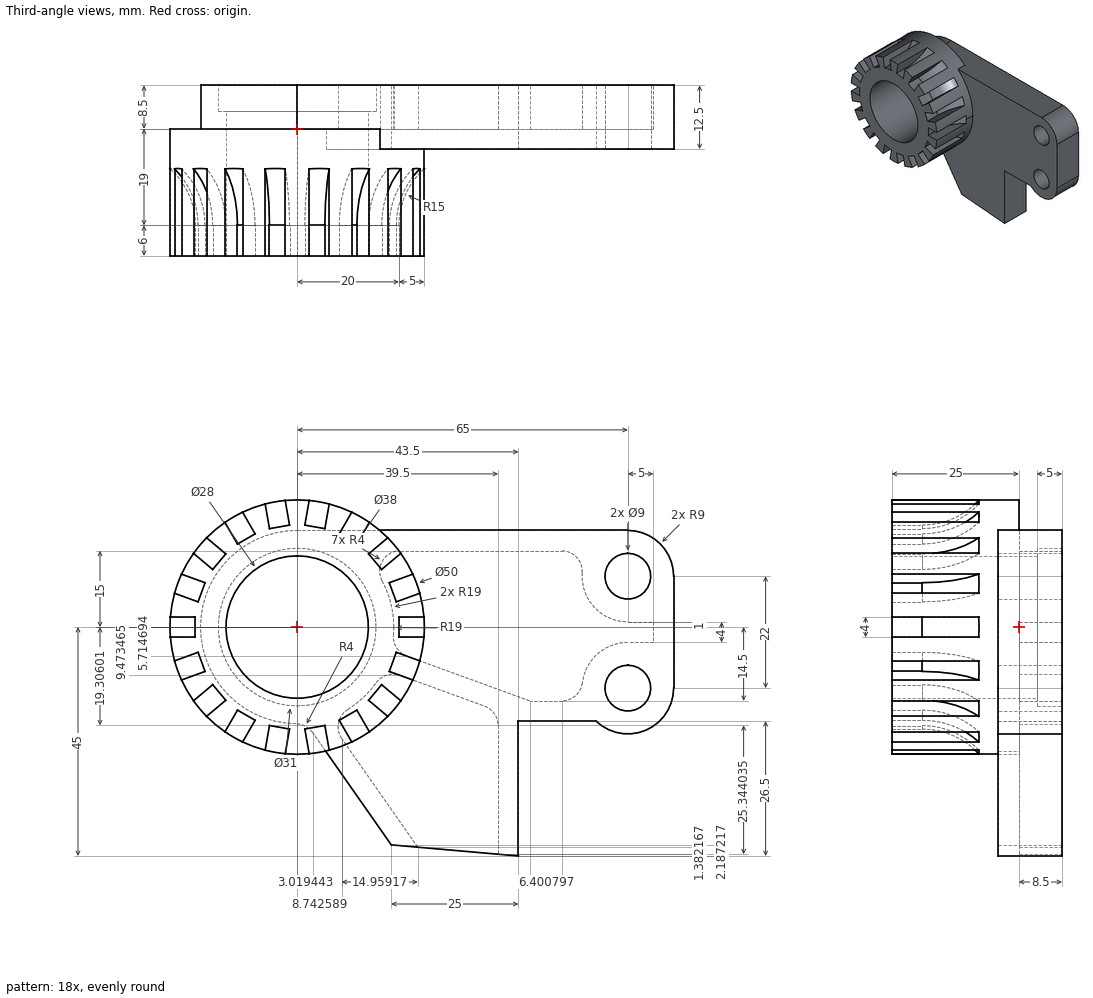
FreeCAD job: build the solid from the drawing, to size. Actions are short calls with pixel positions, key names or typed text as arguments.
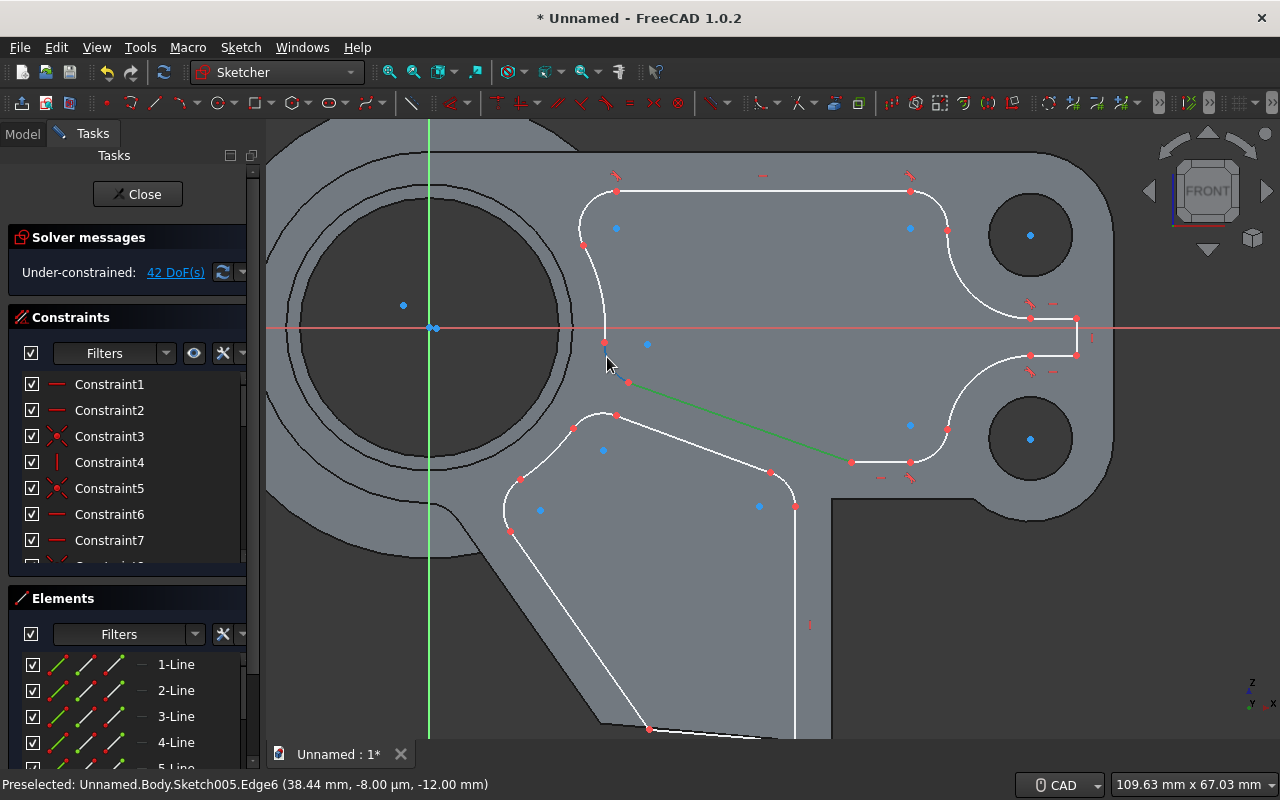
click(607, 357)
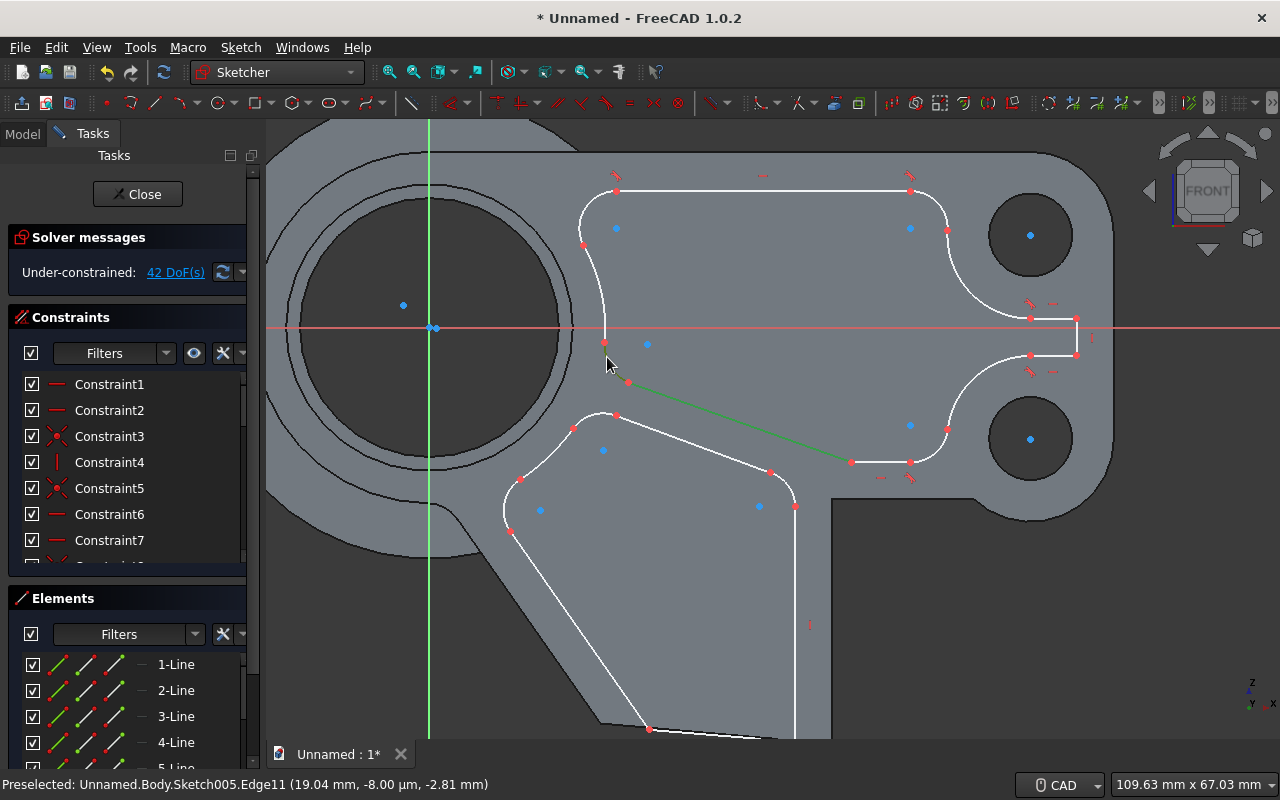
click(606, 104)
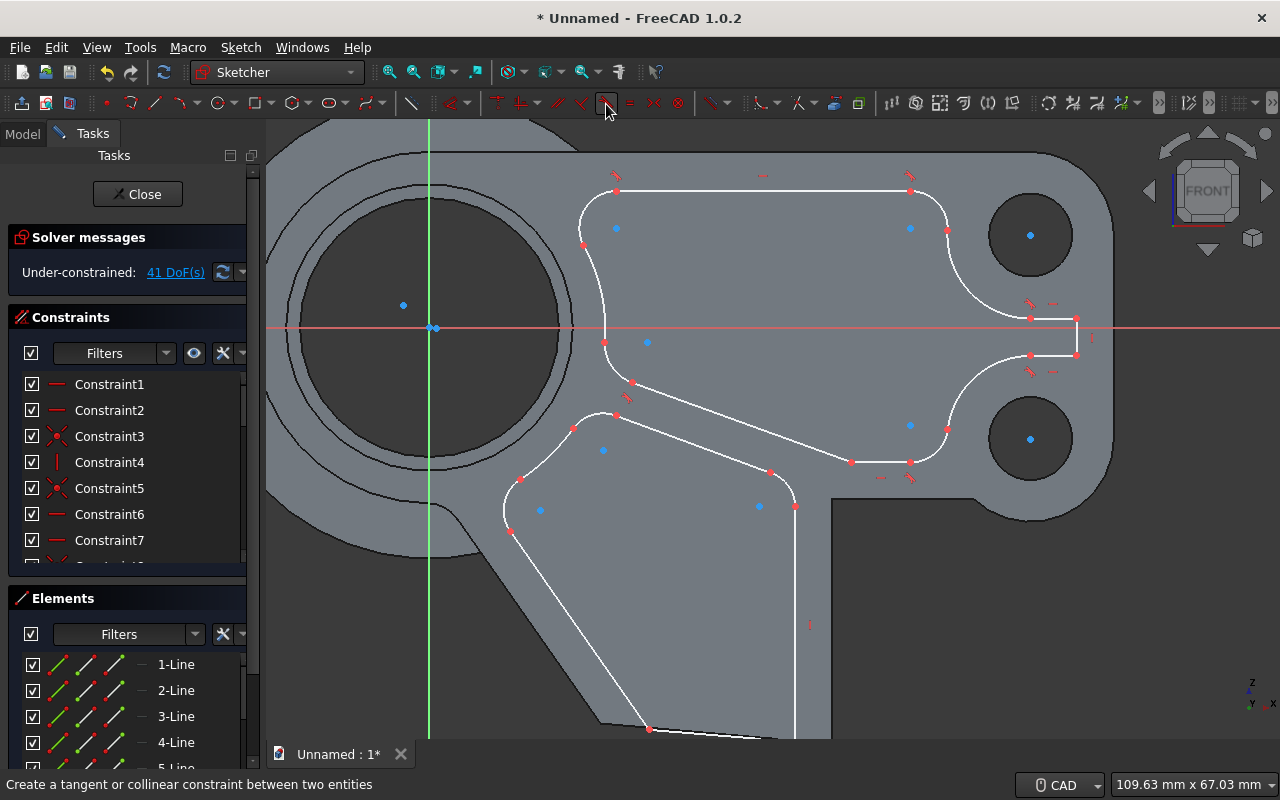
click(944, 213)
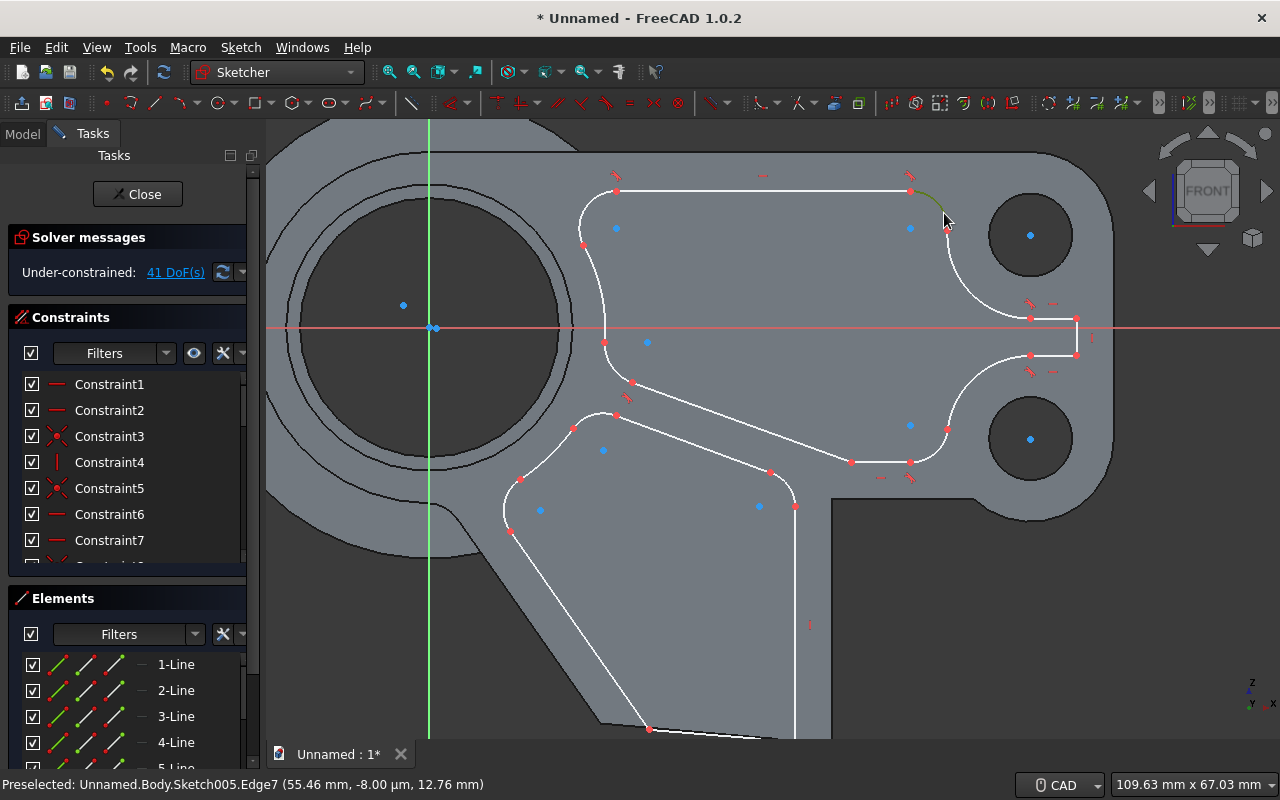
click(955, 270)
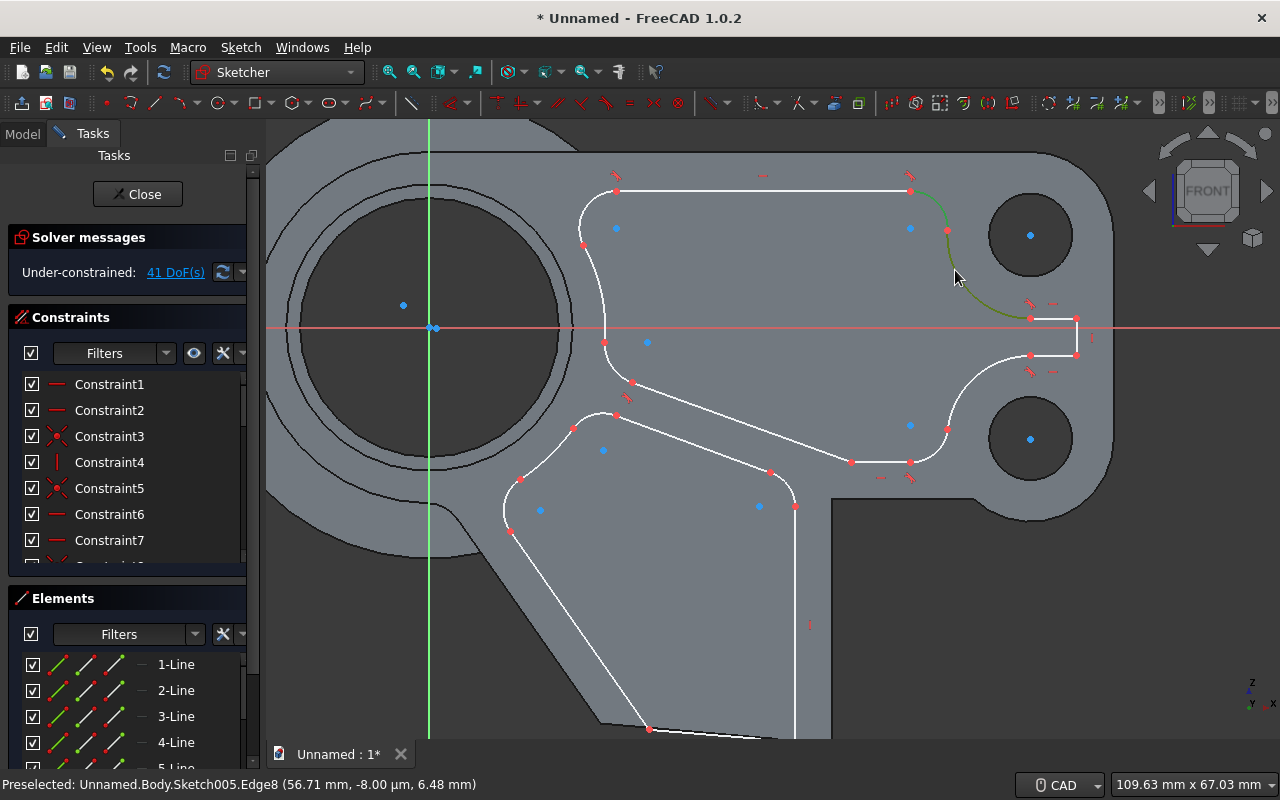
click(606, 104)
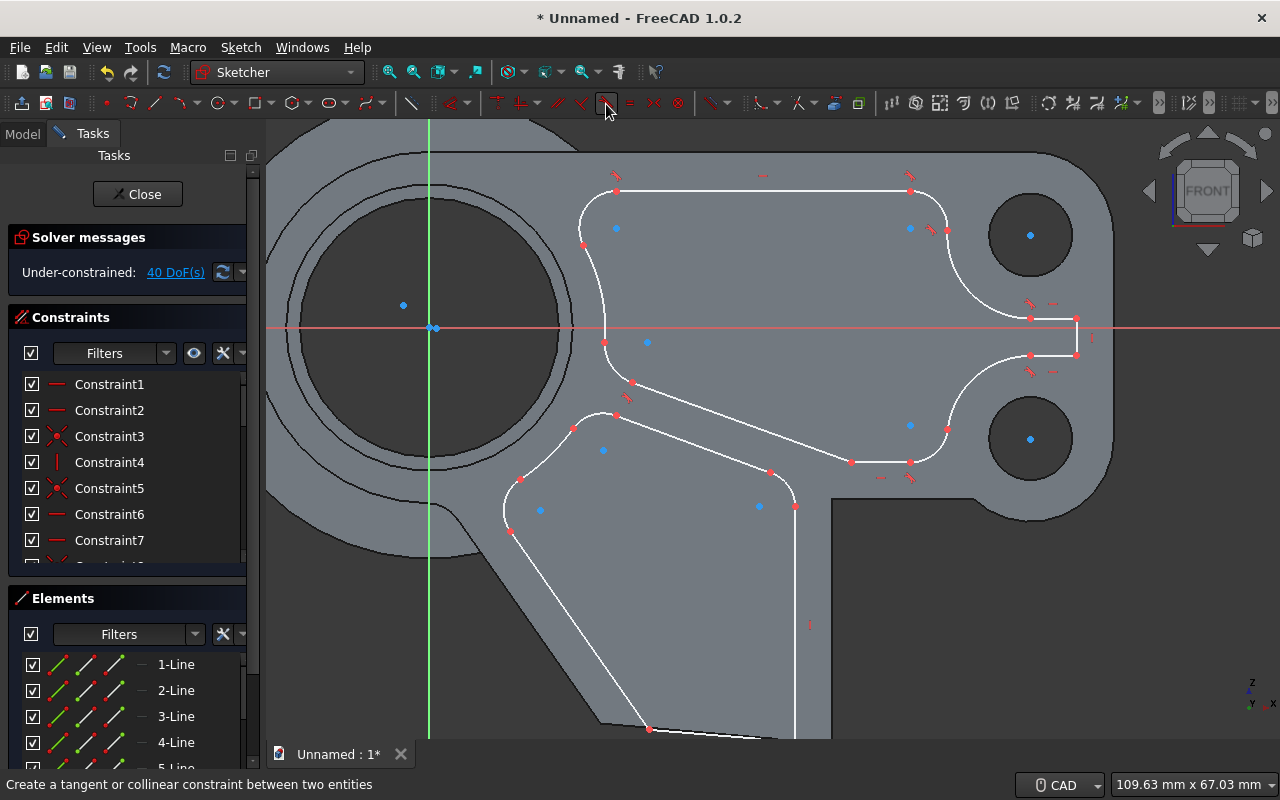
click(996, 364)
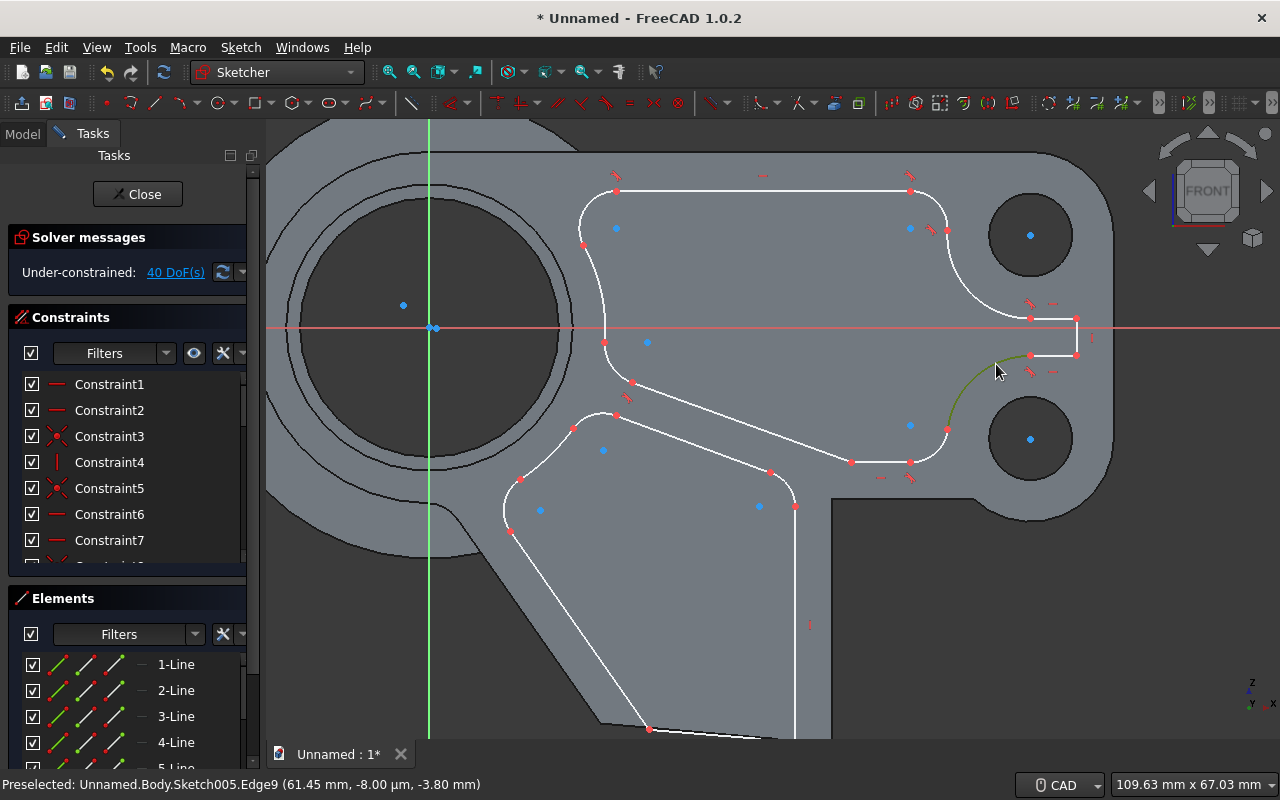
click(927, 459)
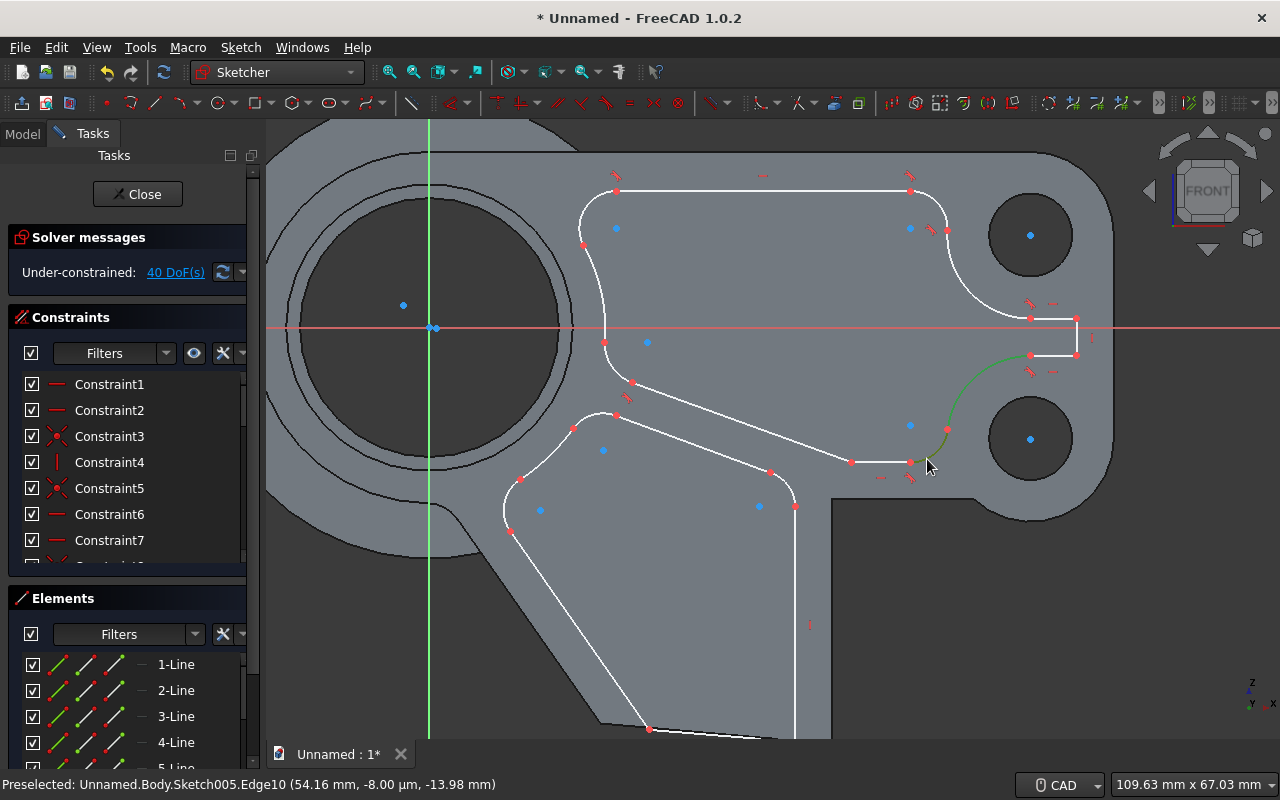
click(606, 104)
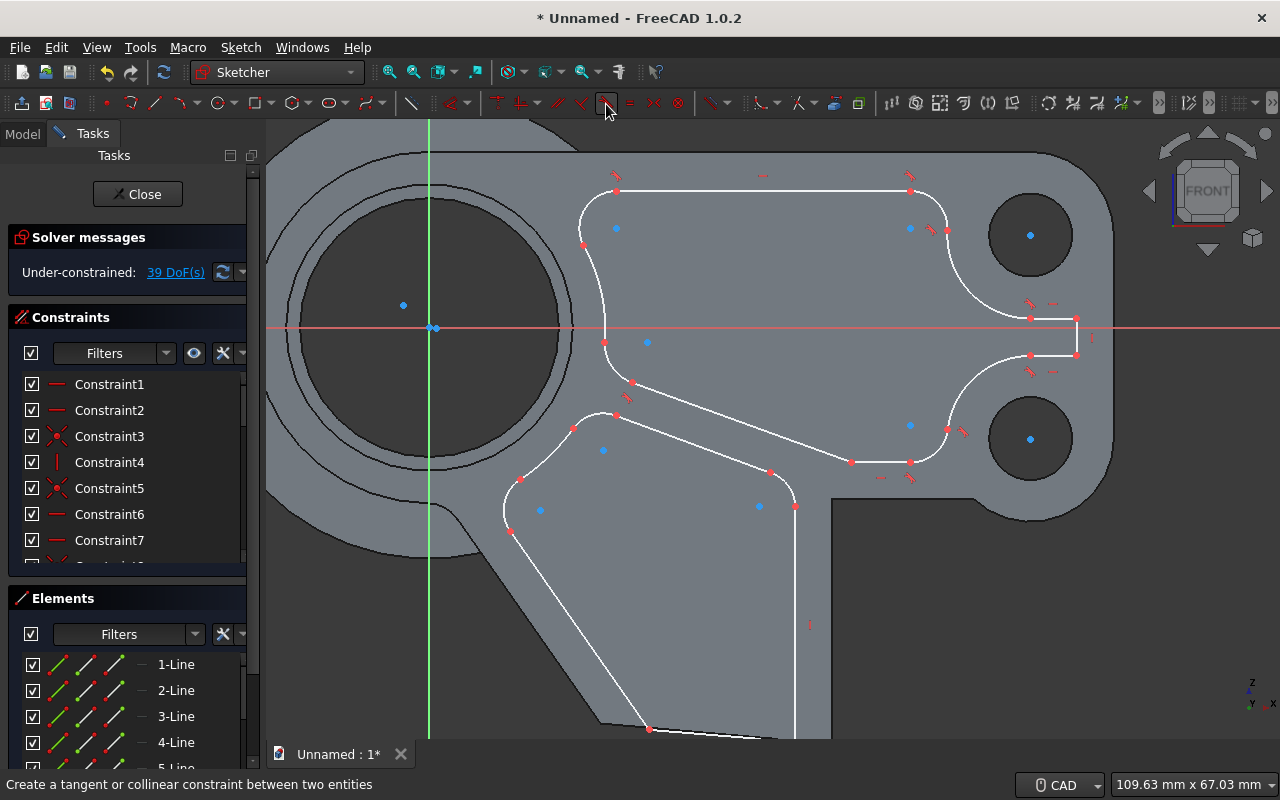
click(607, 358)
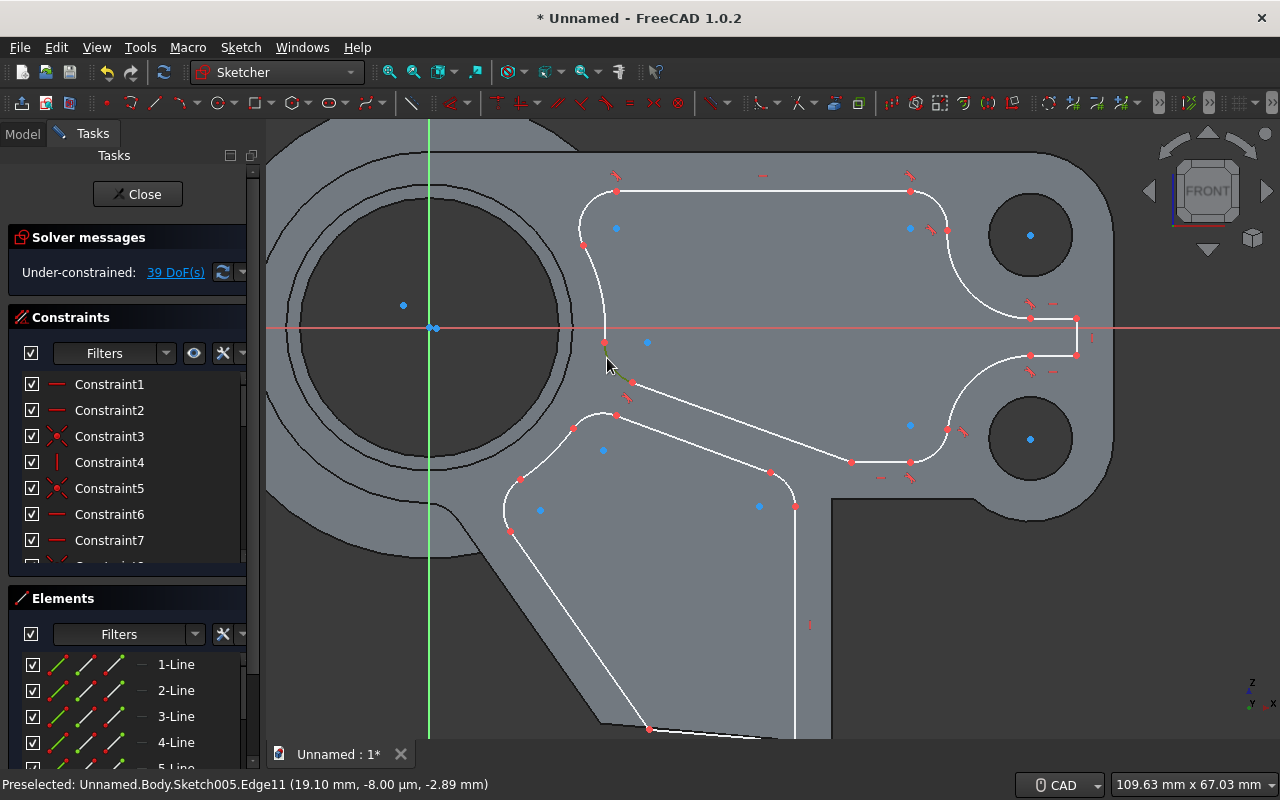
click(604, 313)